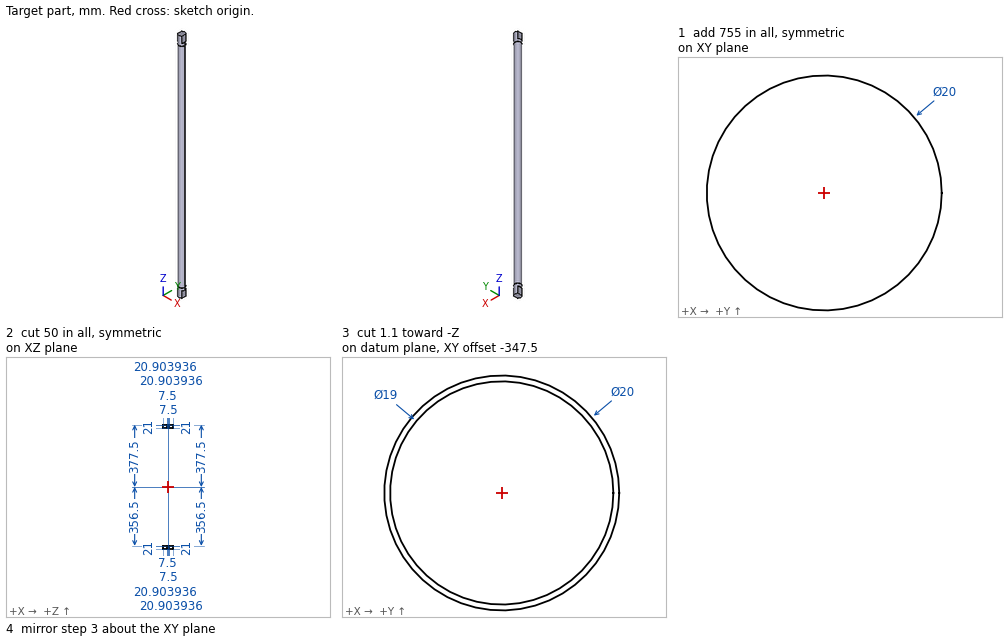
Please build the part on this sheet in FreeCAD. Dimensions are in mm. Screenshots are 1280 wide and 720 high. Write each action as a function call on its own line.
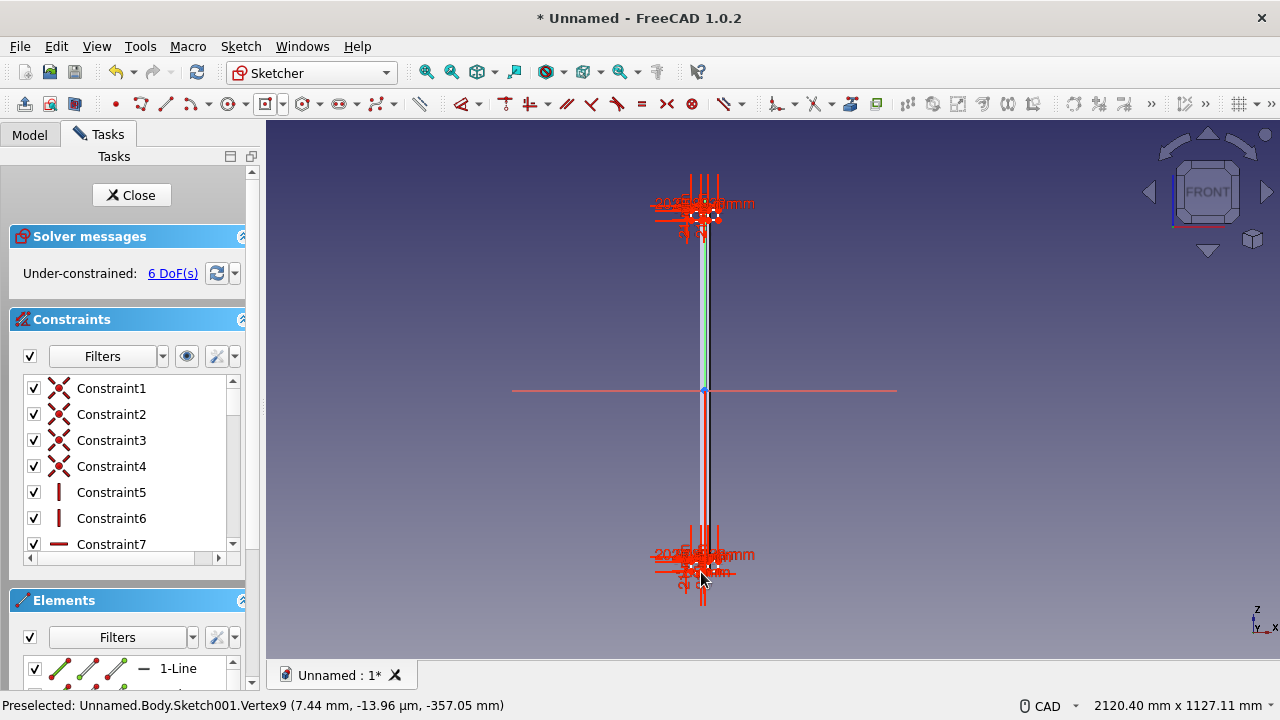
scroll(708, 210, up, 13)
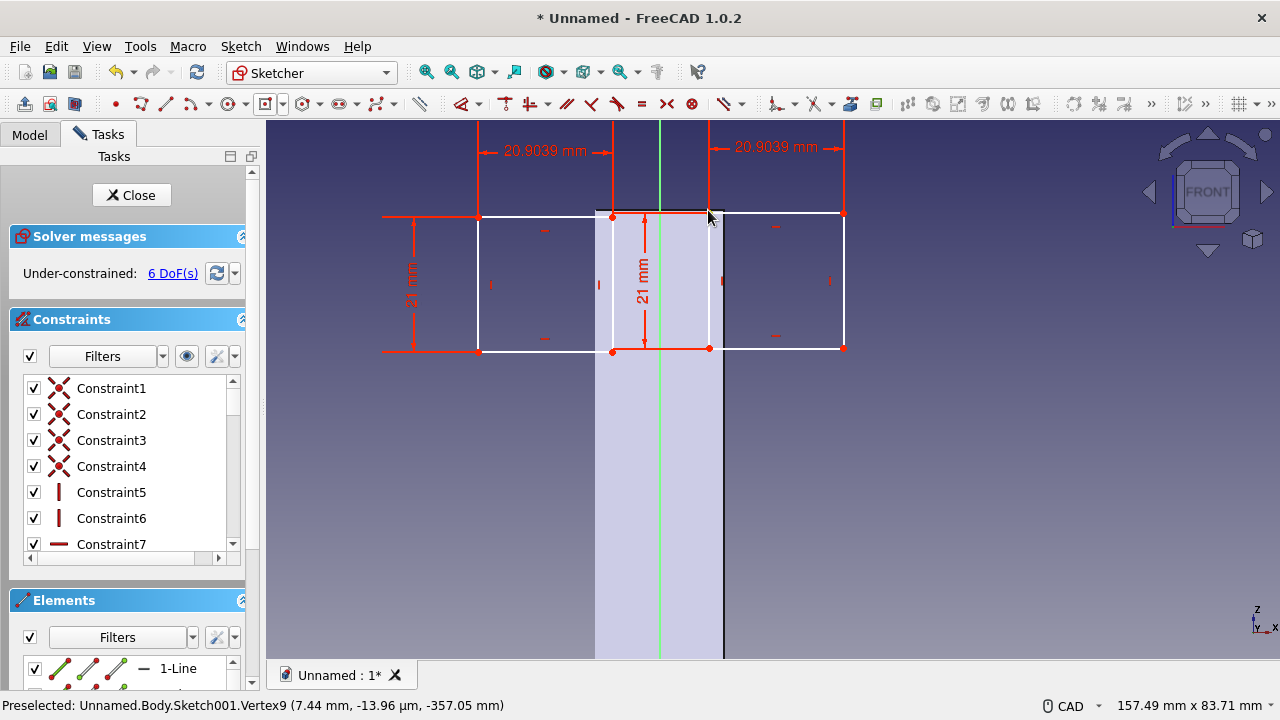
click(709, 213)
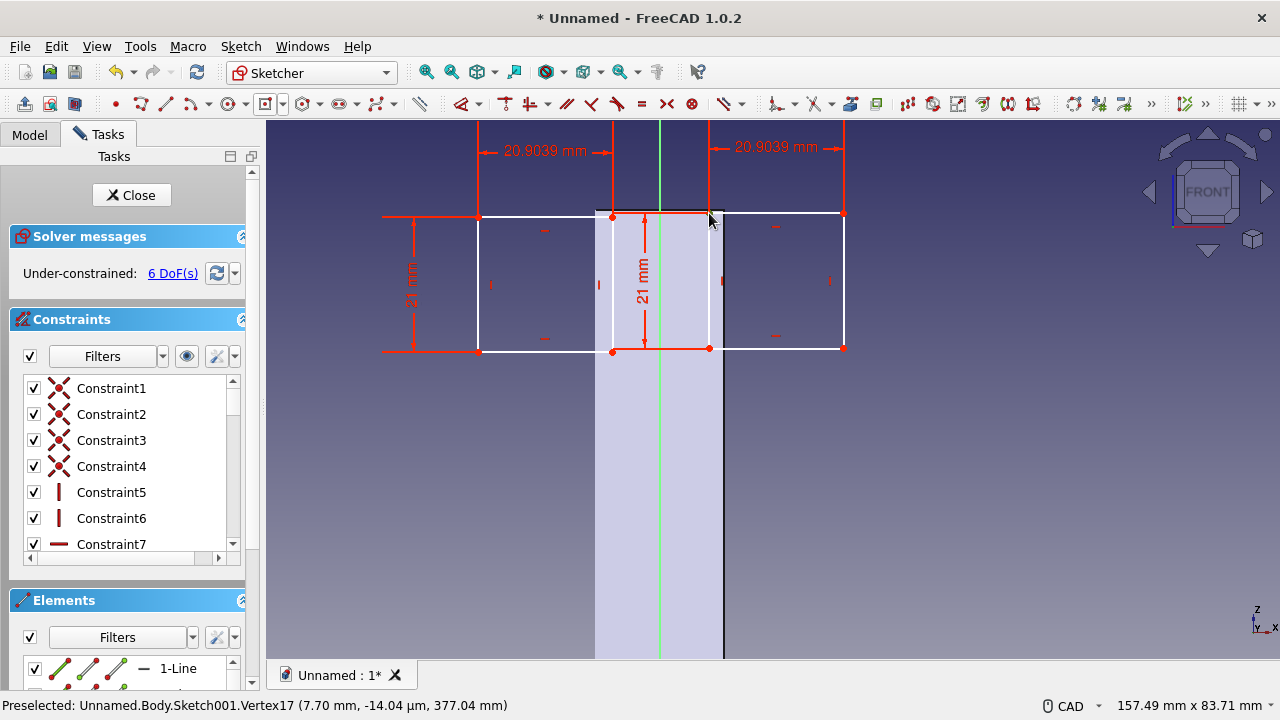
key(l)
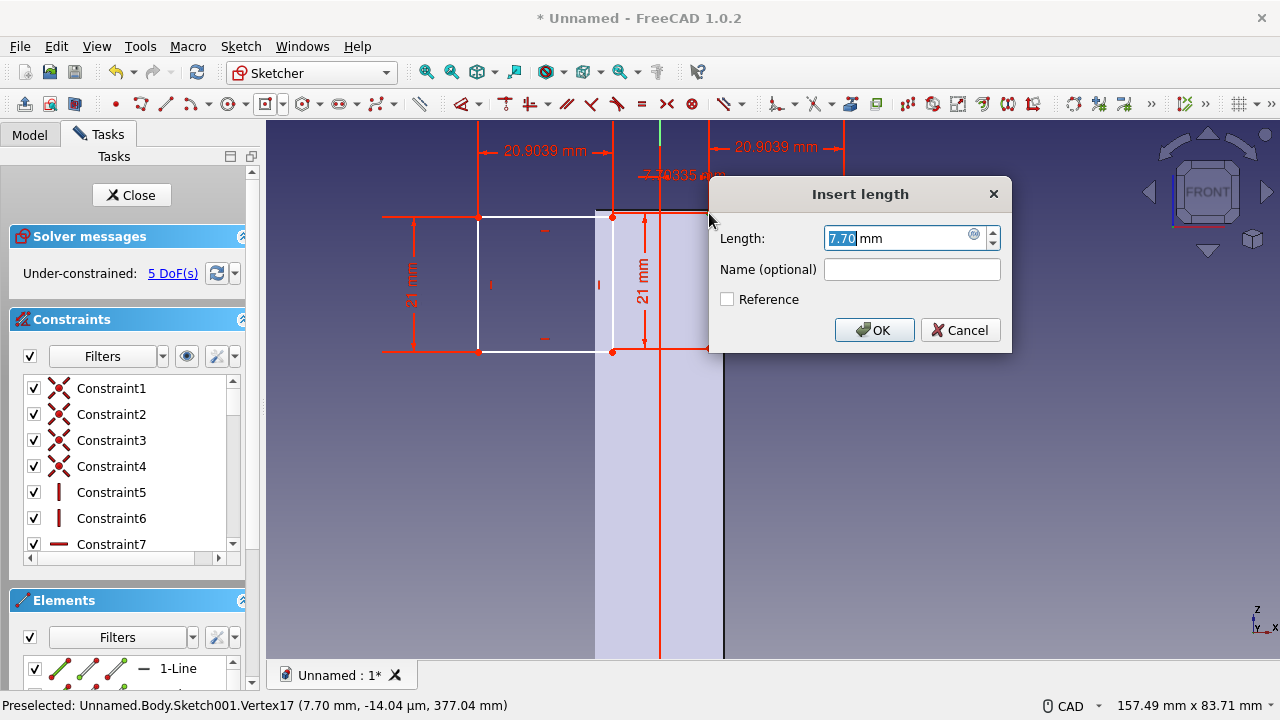
text(7.5)
key(Return)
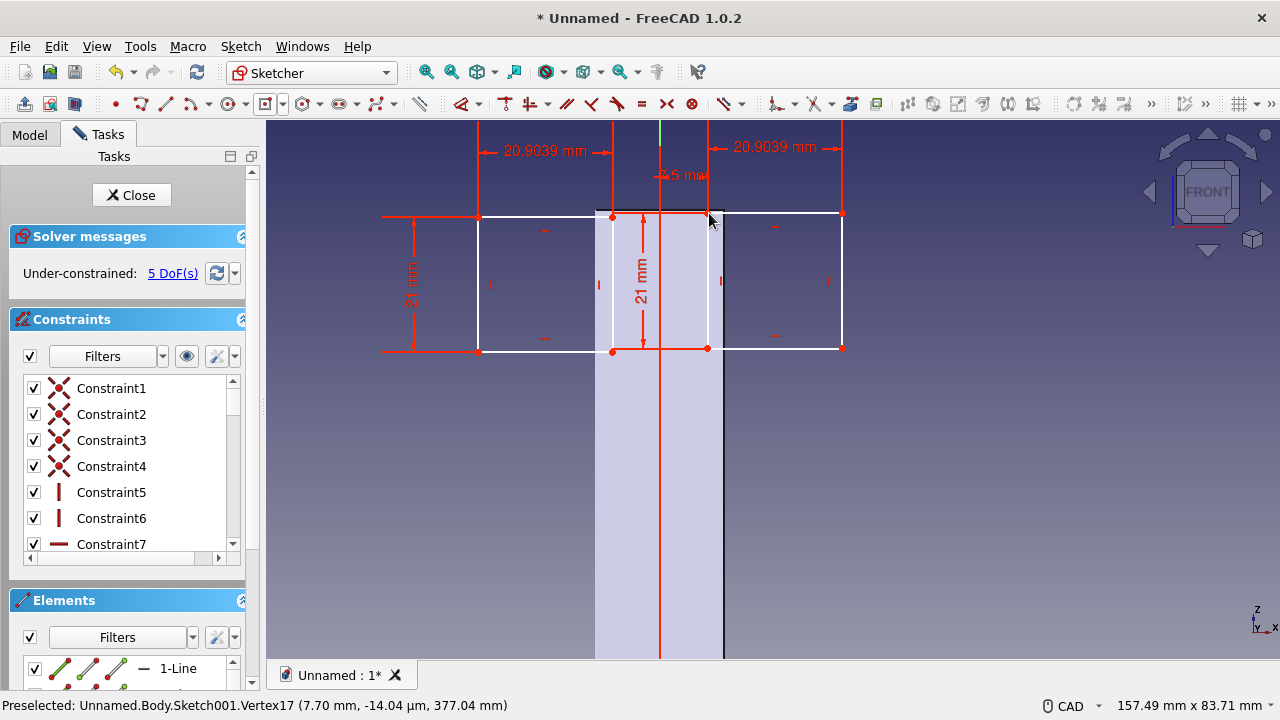
click(613, 352)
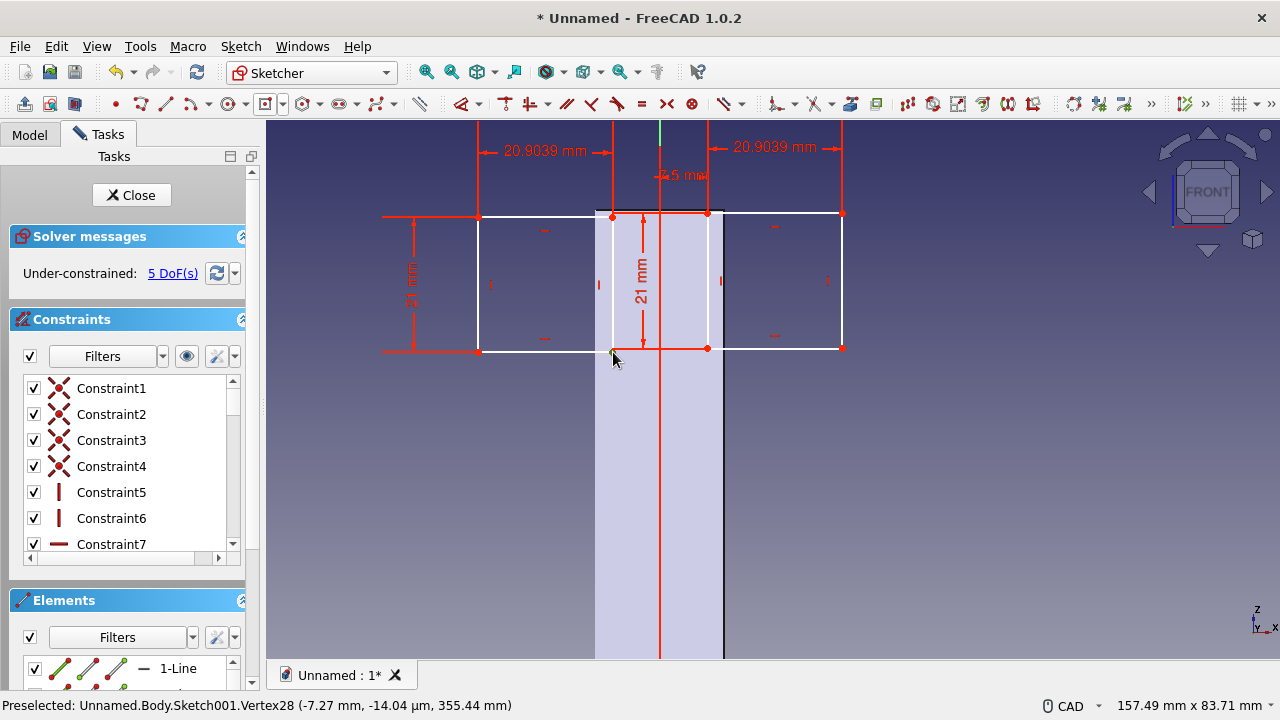
key(l)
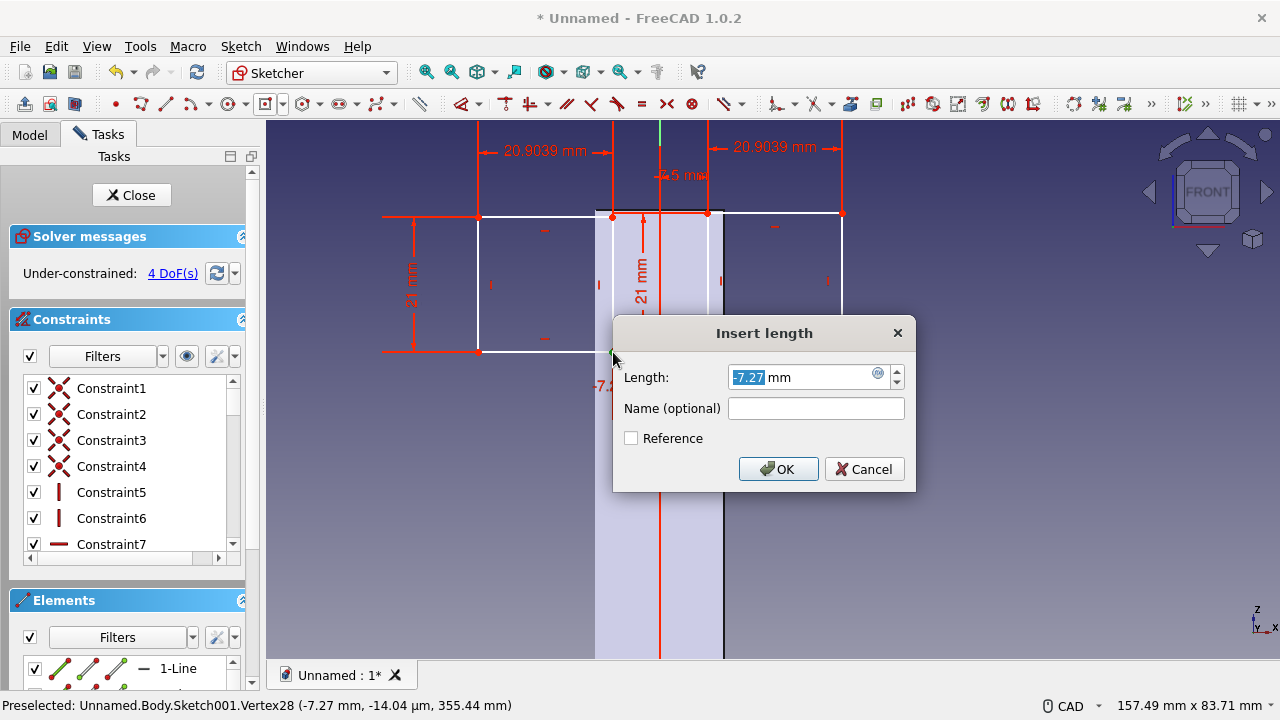
text(-7.5)
key(Return)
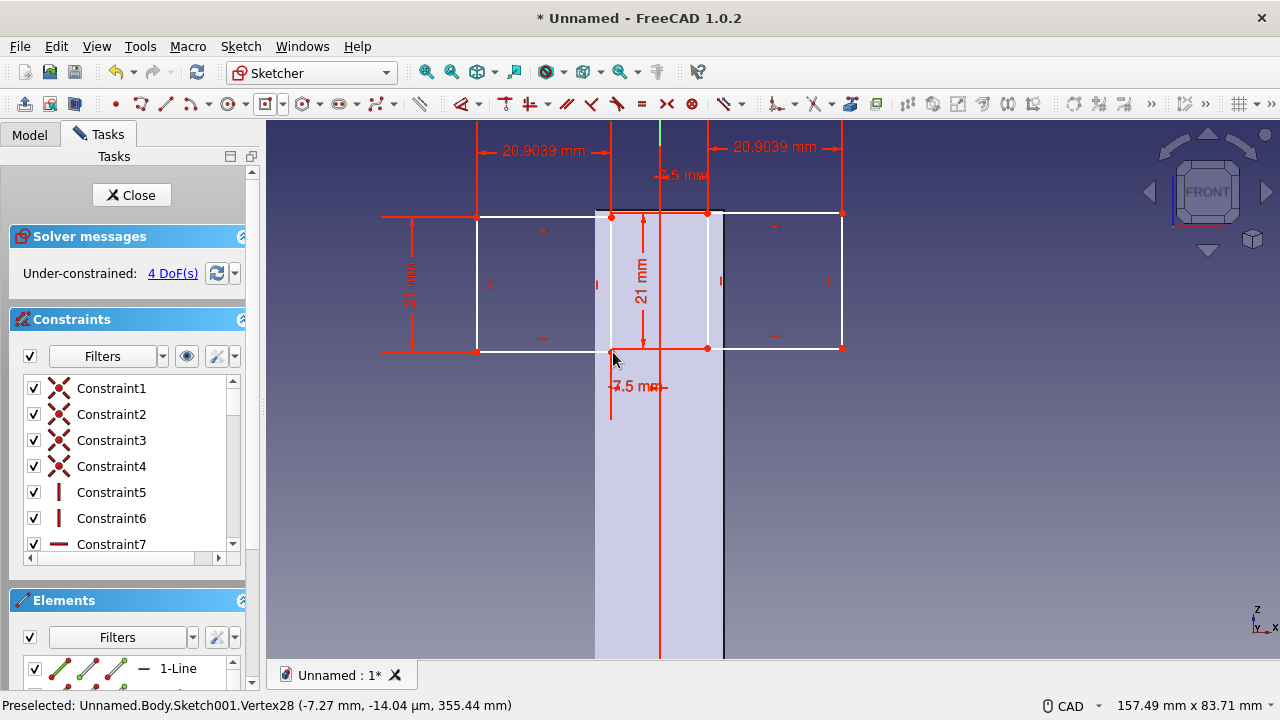
scroll(708, 209, down, 13)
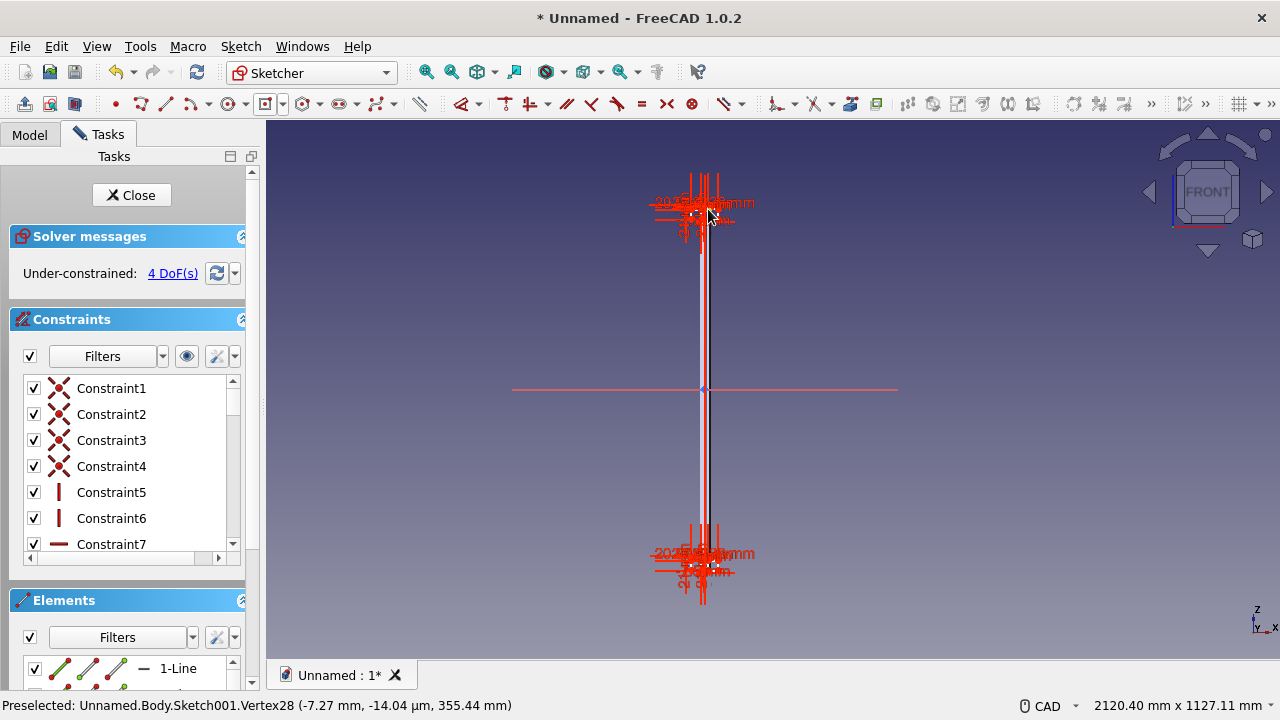
scroll(691, 561, up, 2)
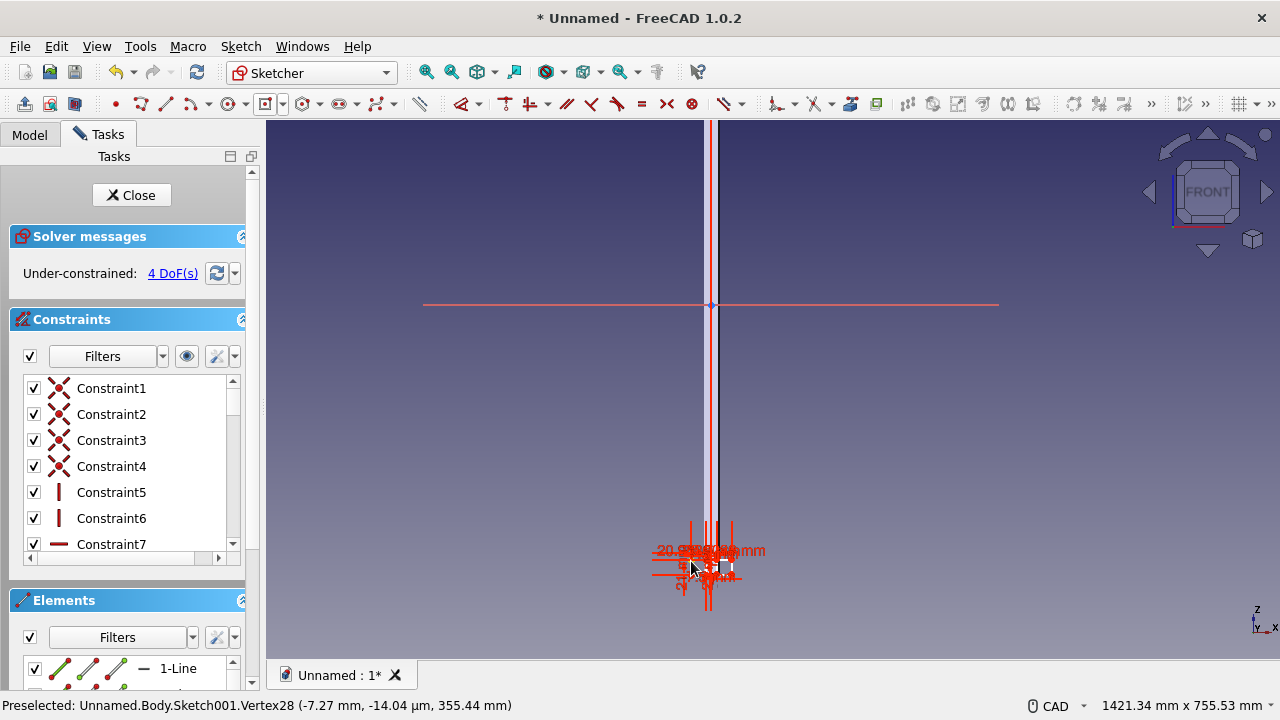
click(691, 560)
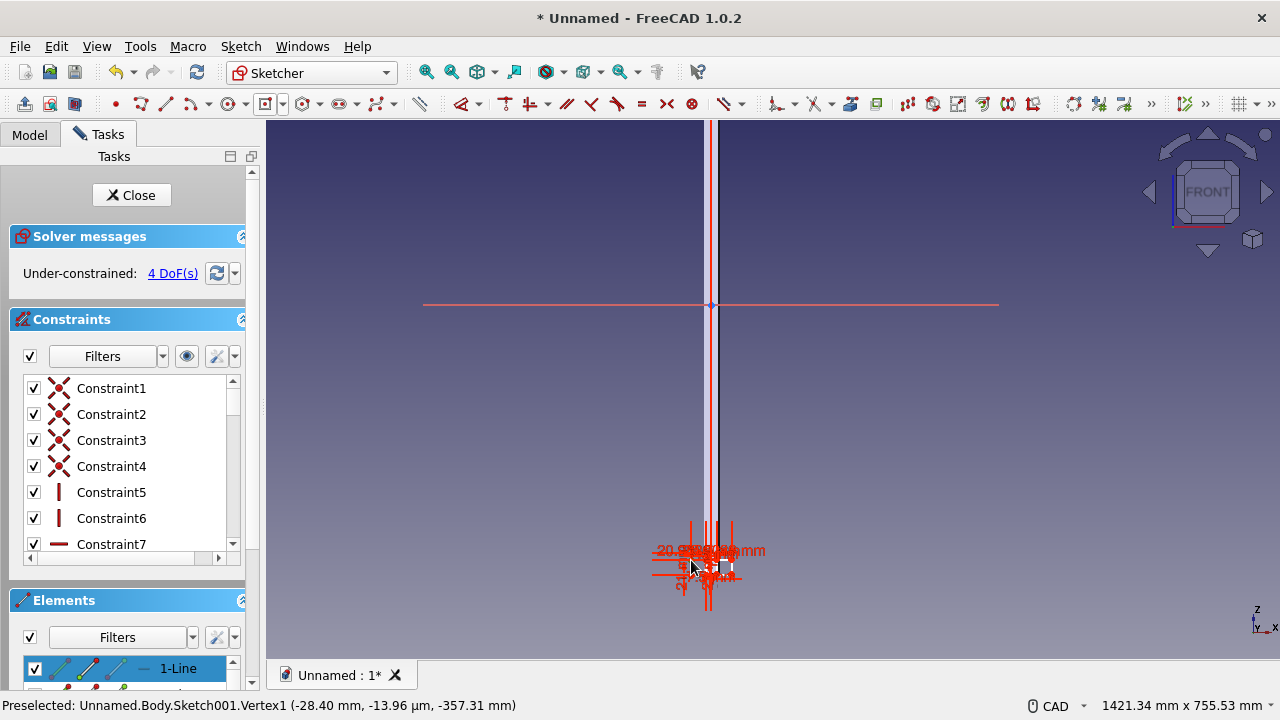
key(i)